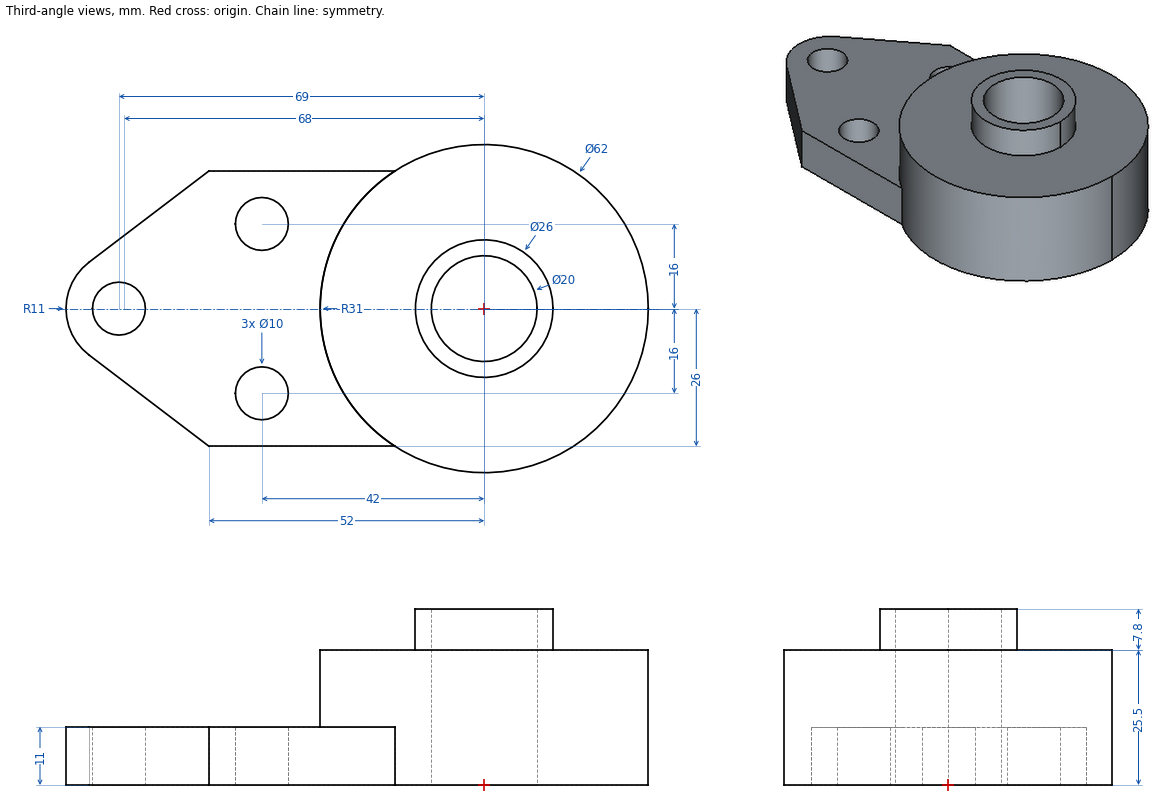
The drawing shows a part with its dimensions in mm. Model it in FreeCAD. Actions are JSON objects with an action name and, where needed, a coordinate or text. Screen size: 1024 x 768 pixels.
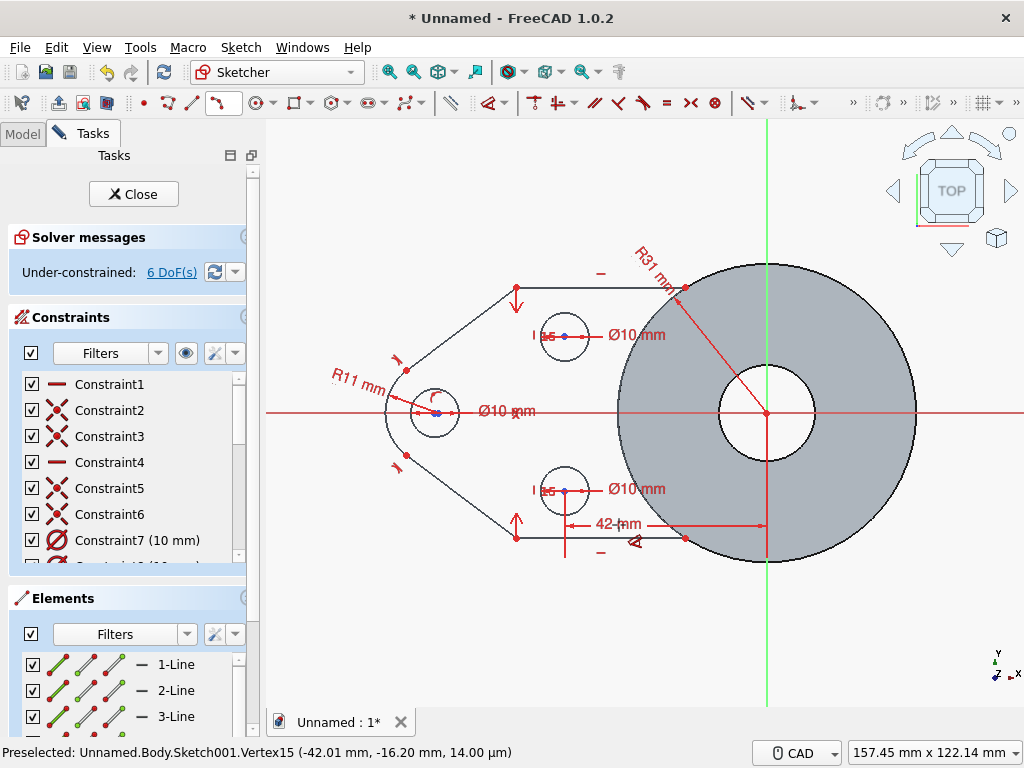
{"action": "left_click", "coordinate": [565, 491]}
{"action": "left_click", "coordinate": [801, 452]}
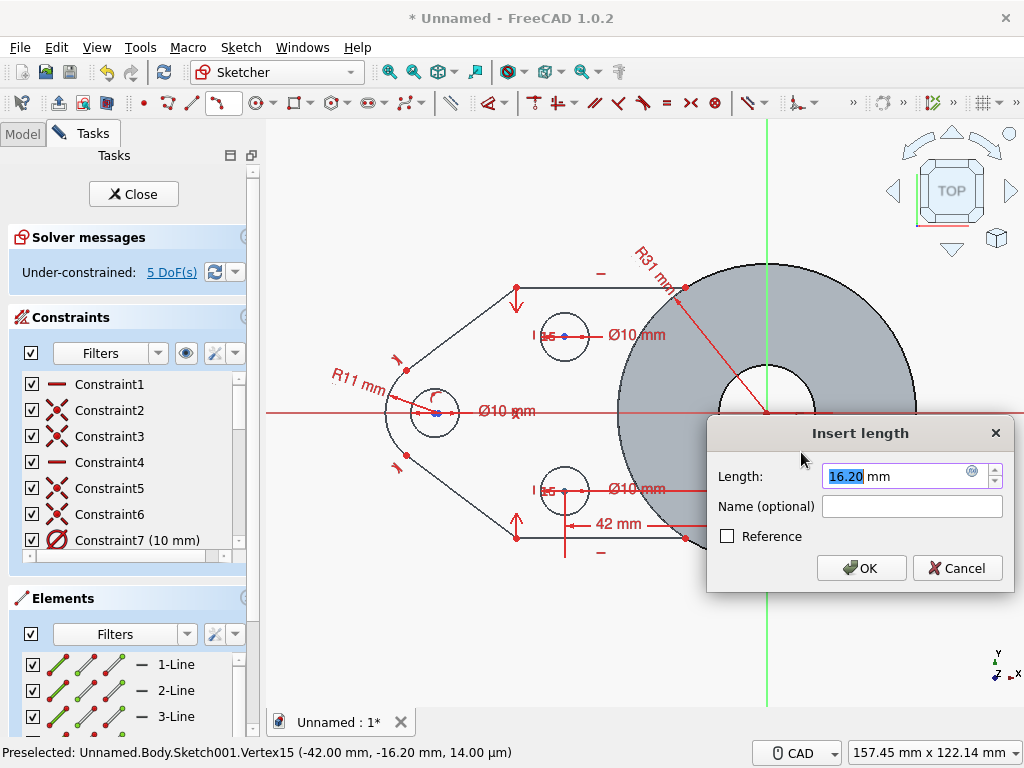
{"action": "type", "text": "16"}
{"action": "key", "text": "Return"}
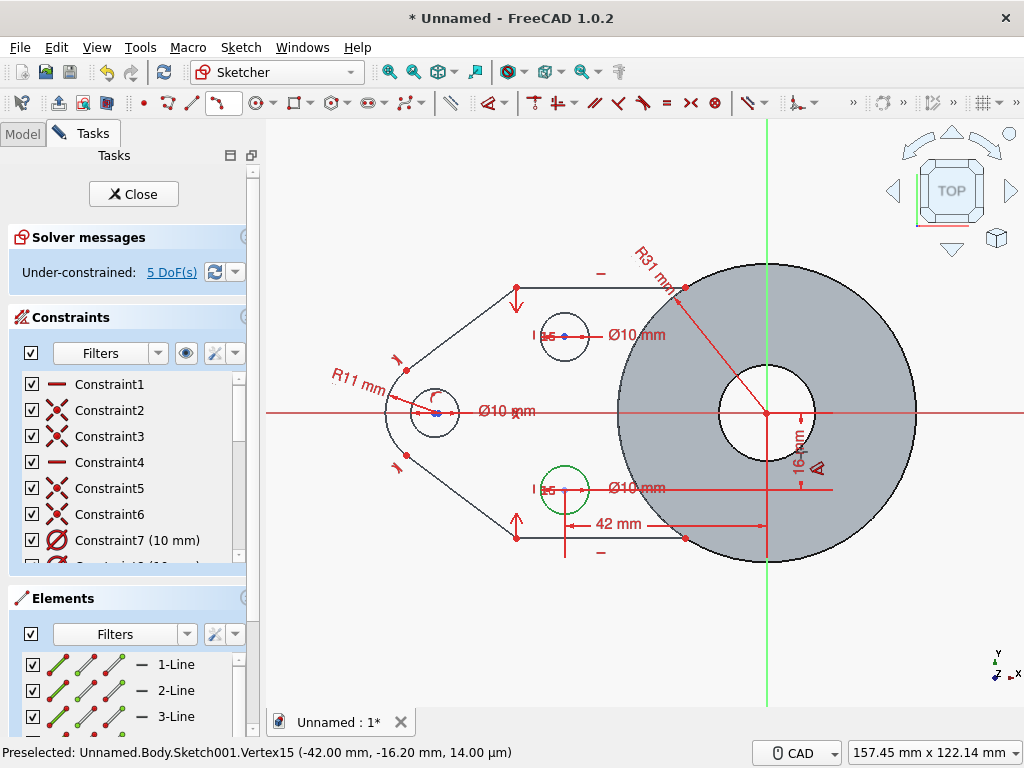
{"action": "scroll", "coordinate": [435, 413], "scroll_direction": "up", "scroll_amount": 7}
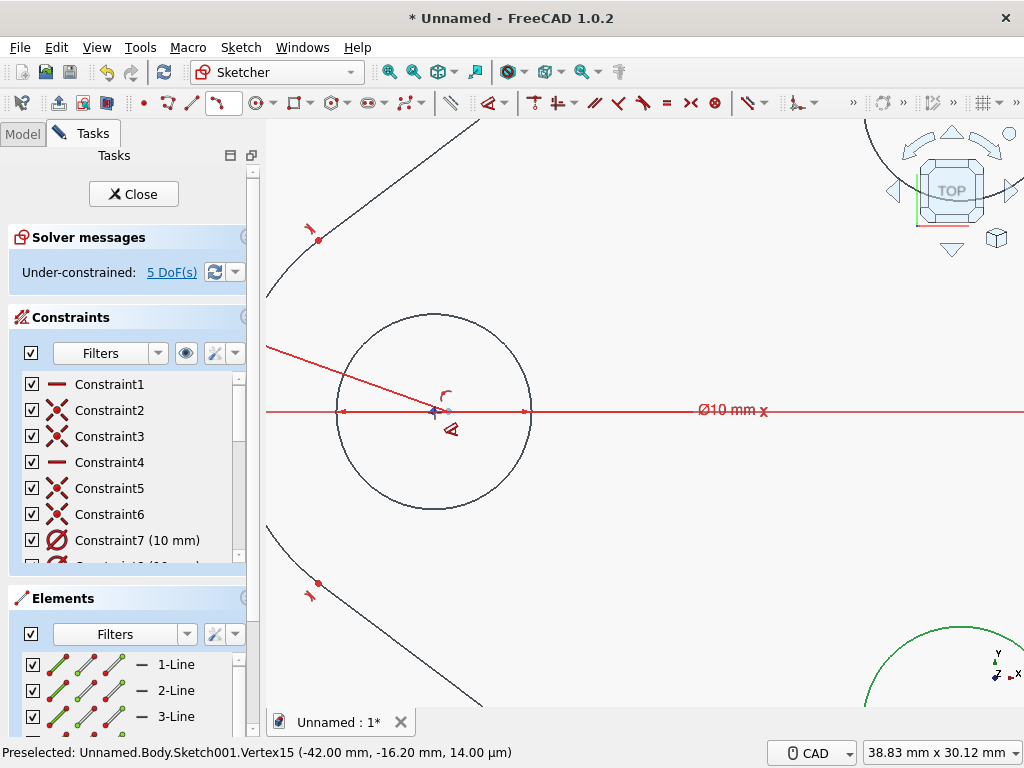
{"action": "left_click", "coordinate": [434, 412]}
{"action": "left_click", "coordinate": [646, 446]}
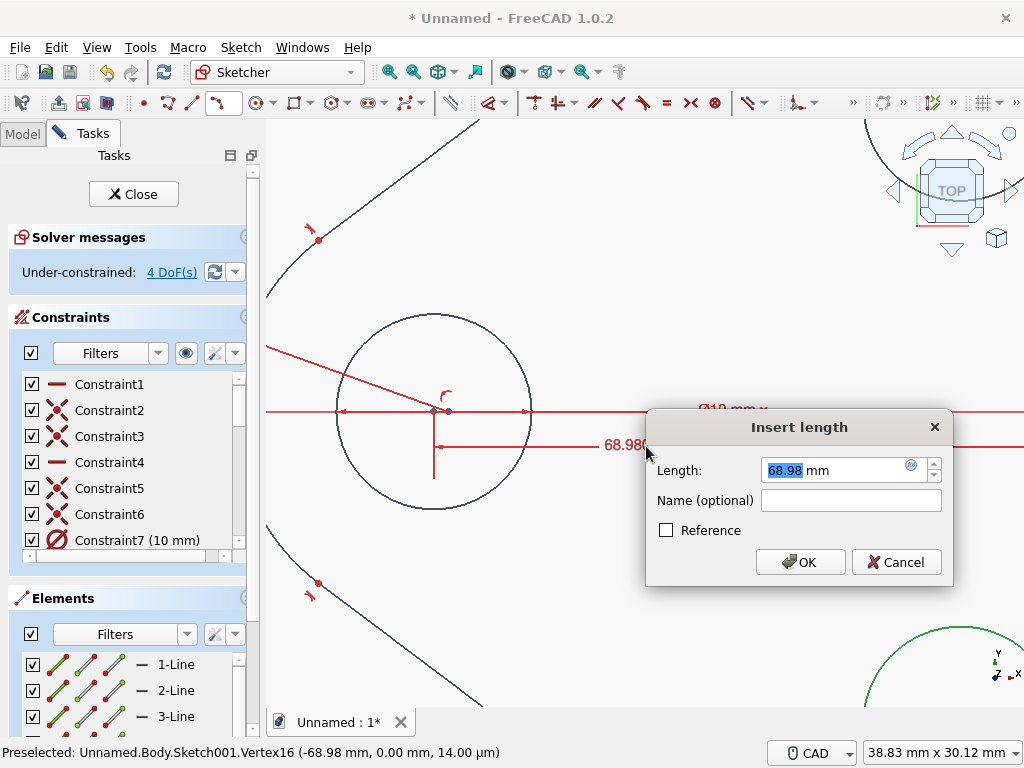
{"action": "type", "text": "69"}
{"action": "key", "text": "Return"}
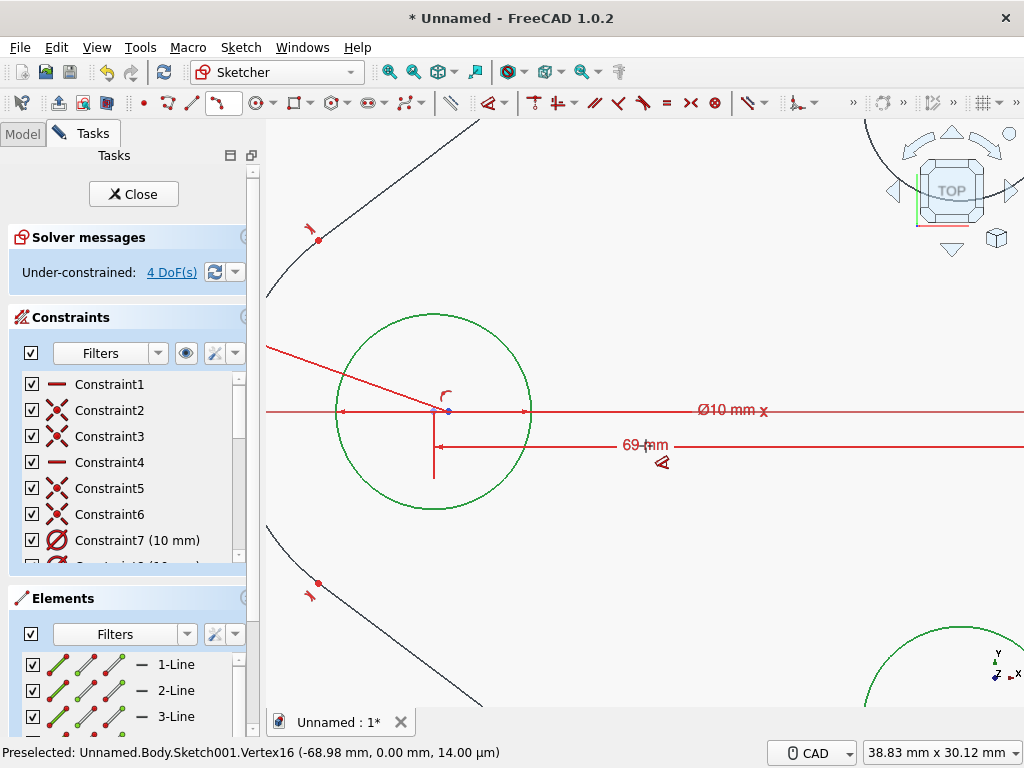
{"action": "scroll", "coordinate": [435, 413], "scroll_direction": "down", "scroll_amount": 7}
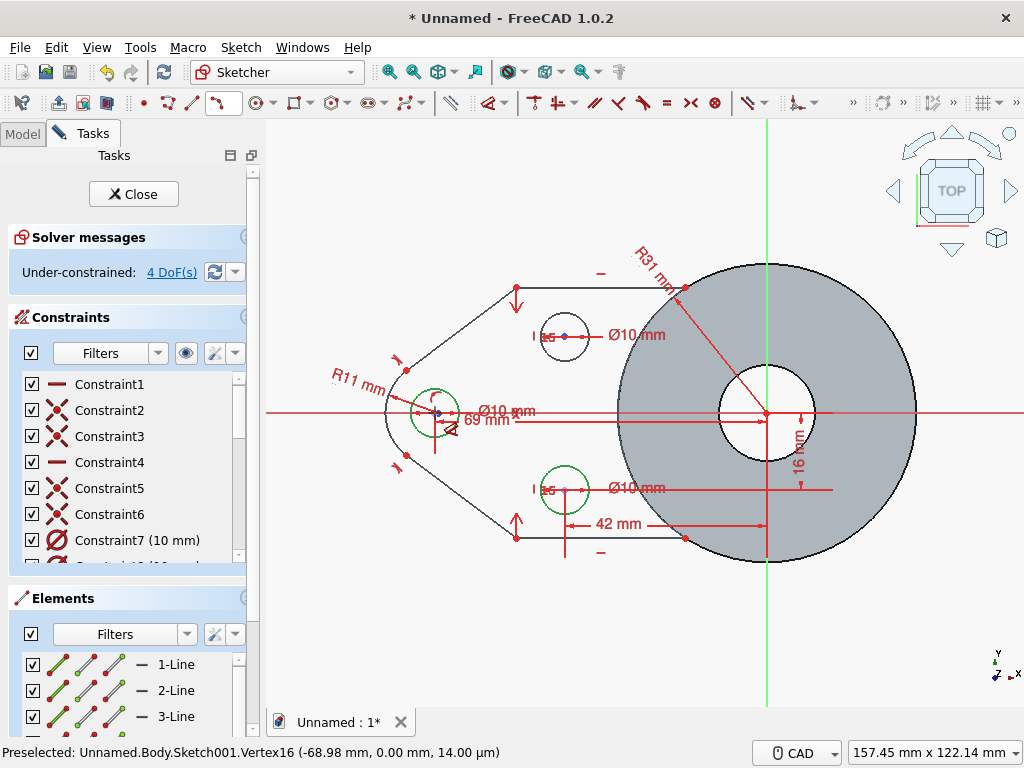
{"action": "left_click", "coordinate": [565, 337]}
{"action": "left_click", "coordinate": [801, 375]}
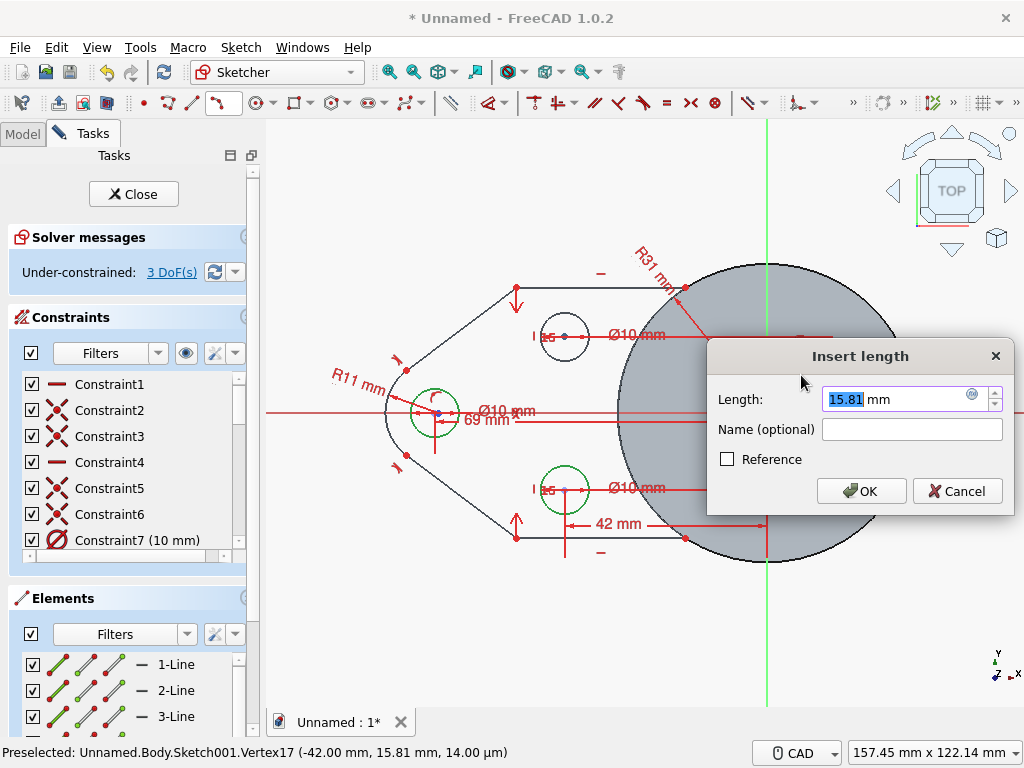
{"action": "type", "text": "16"}
{"action": "key", "text": "Return"}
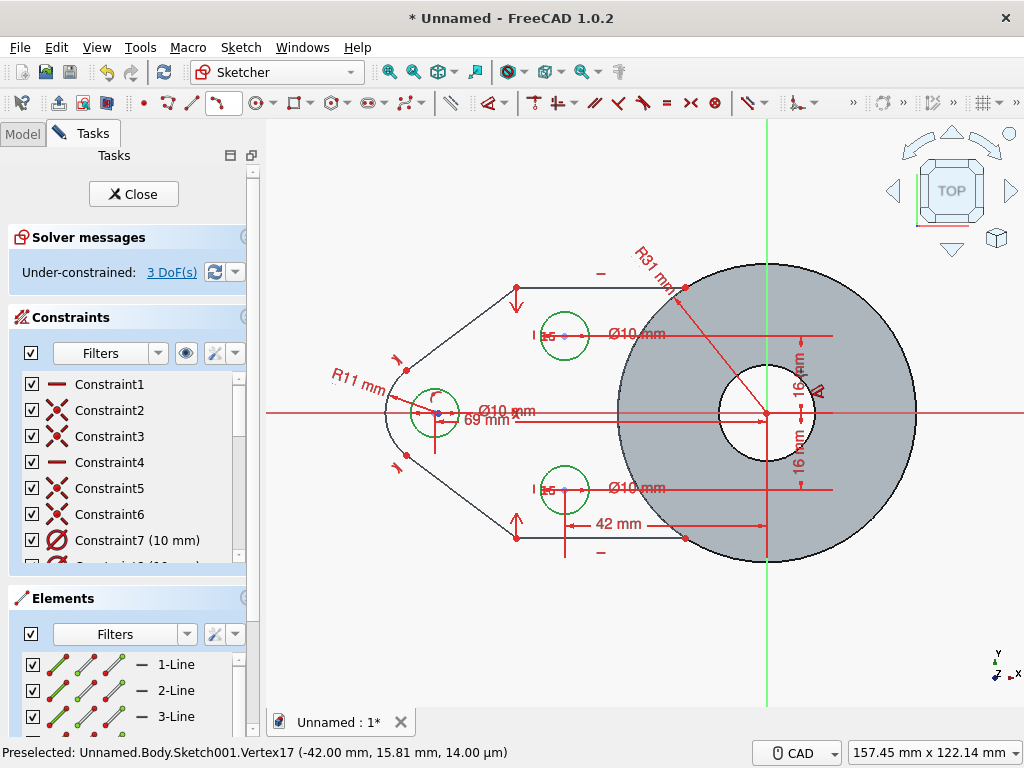
{"action": "left_click", "coordinate": [686, 538]}
{"action": "left_click", "coordinate": [801, 476]}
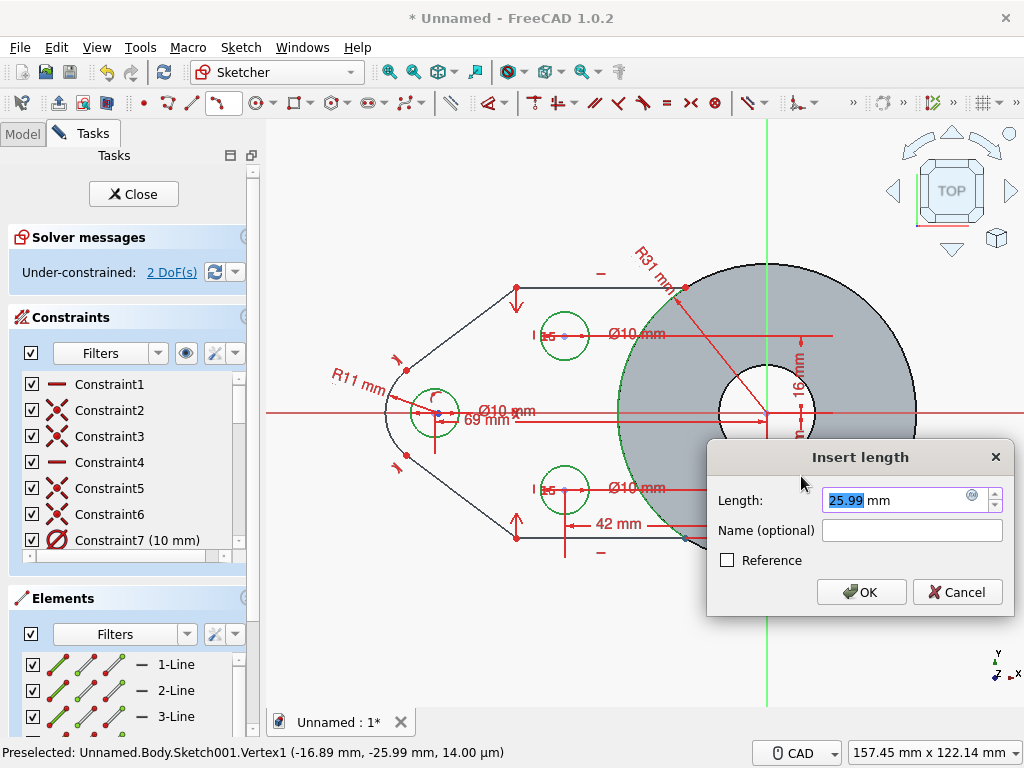
{"action": "type", "text": "26"}
{"action": "key", "text": "Return"}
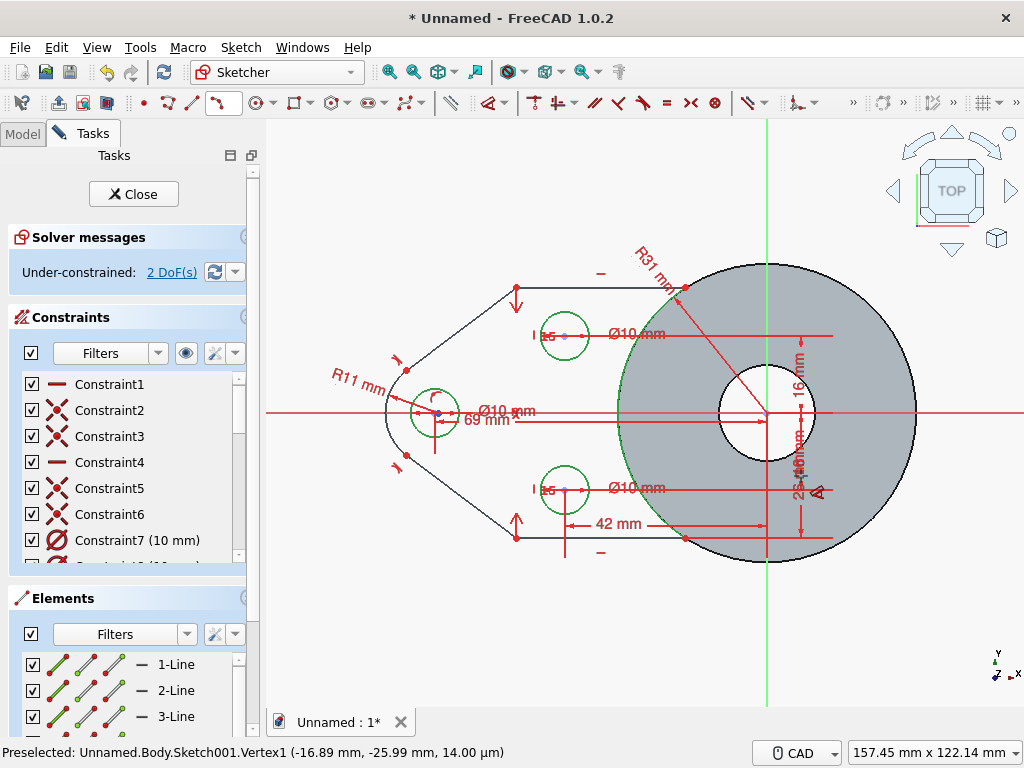
{"action": "left_click", "coordinate": [516, 538]}
{"action": "left_click", "coordinate": [642, 572]}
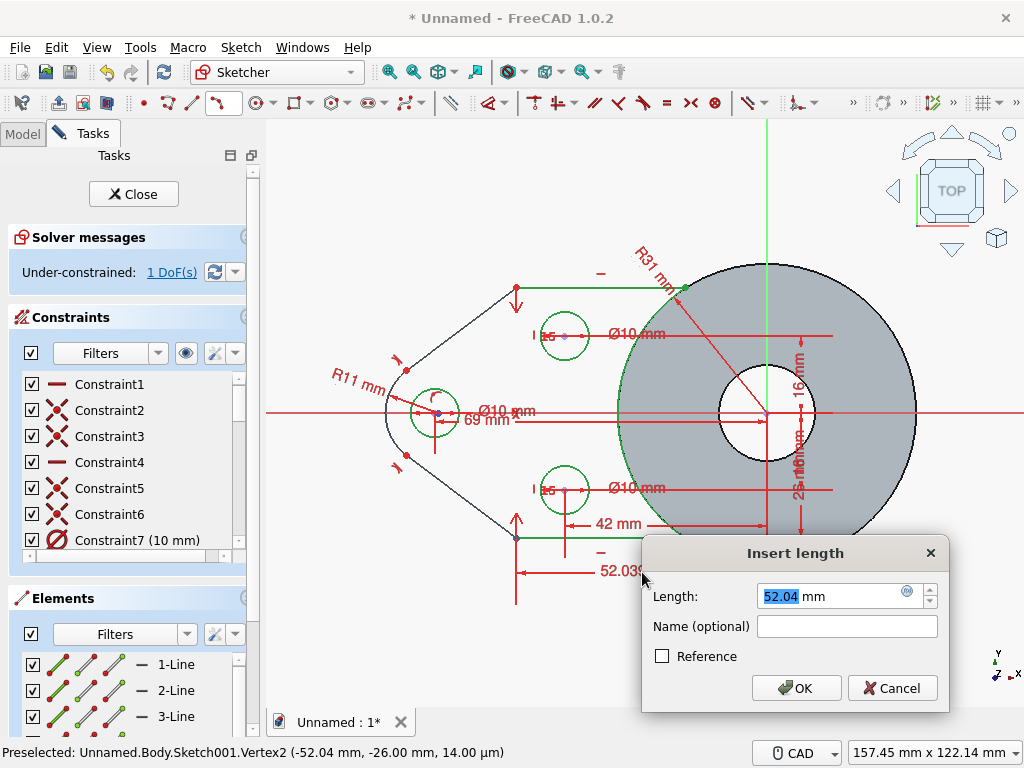
{"action": "type", "text": "52"}
{"action": "key", "text": "Return"}